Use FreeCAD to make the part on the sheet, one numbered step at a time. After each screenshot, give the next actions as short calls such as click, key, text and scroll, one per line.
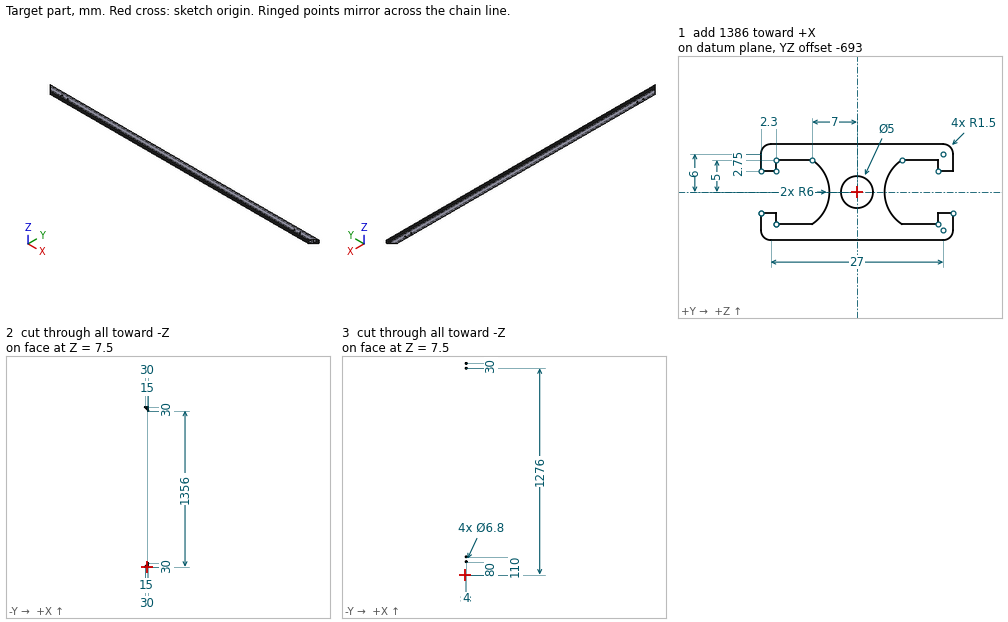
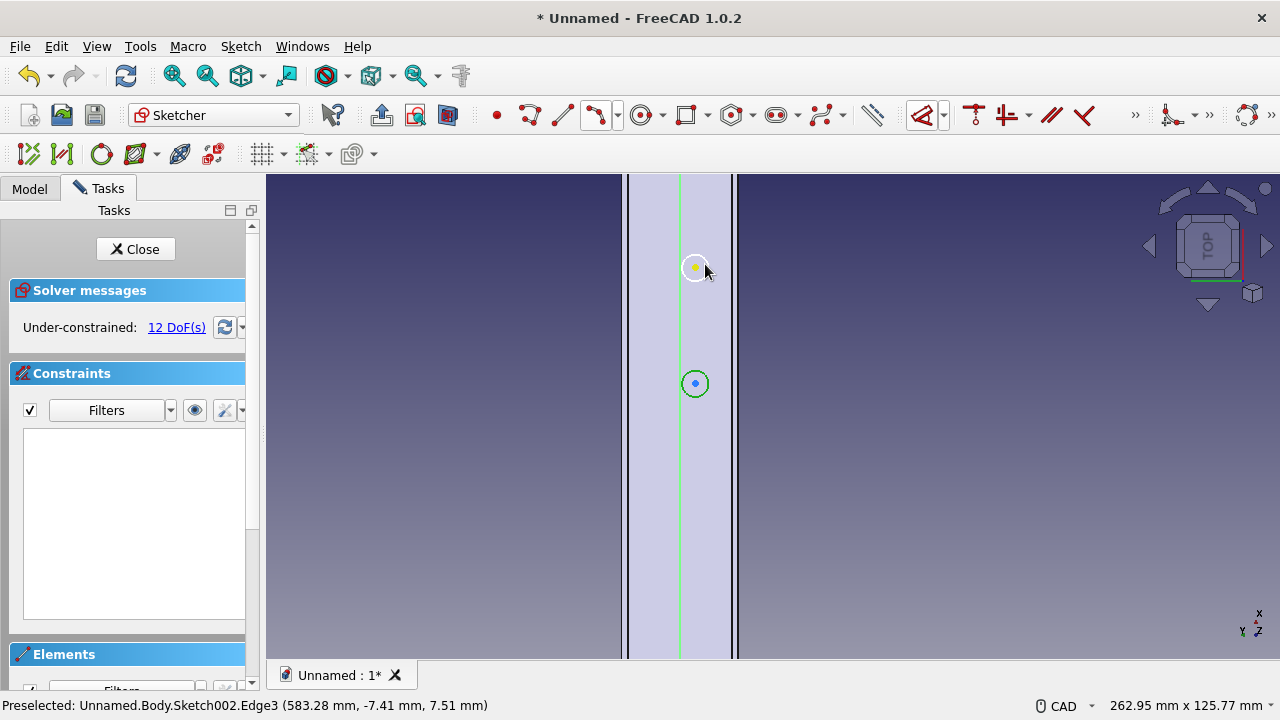
click(705, 259)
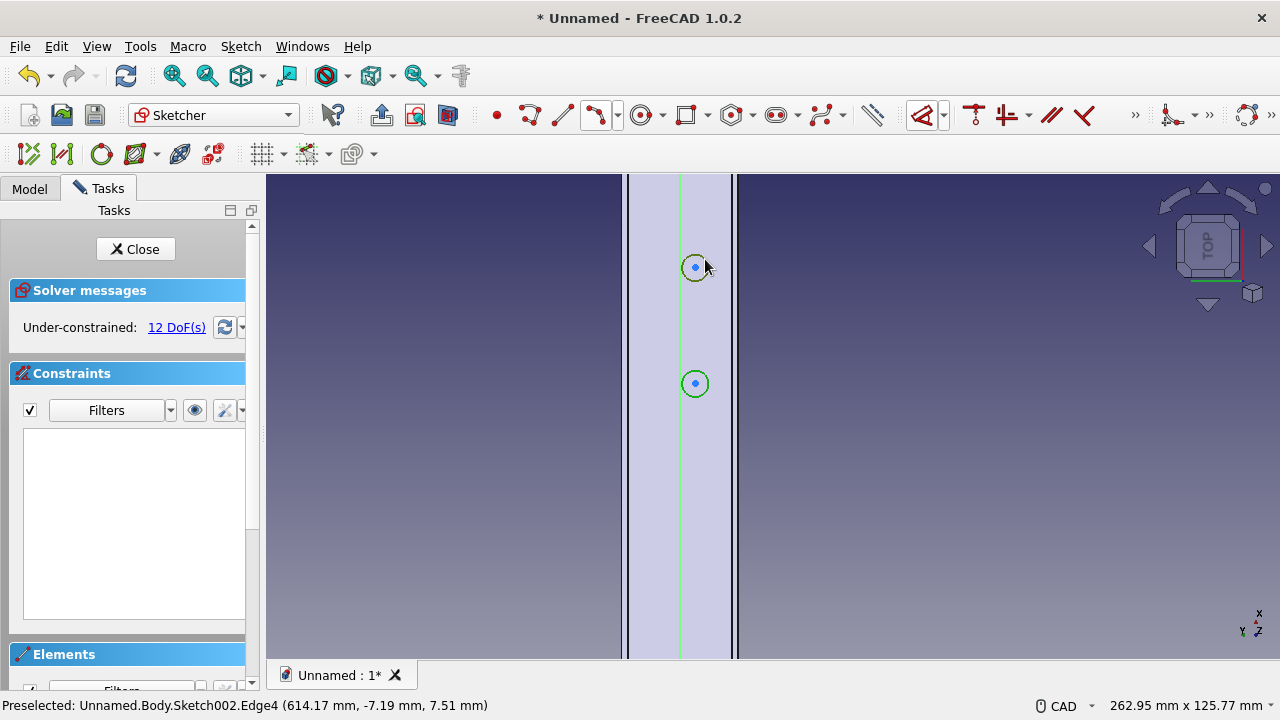
key(e)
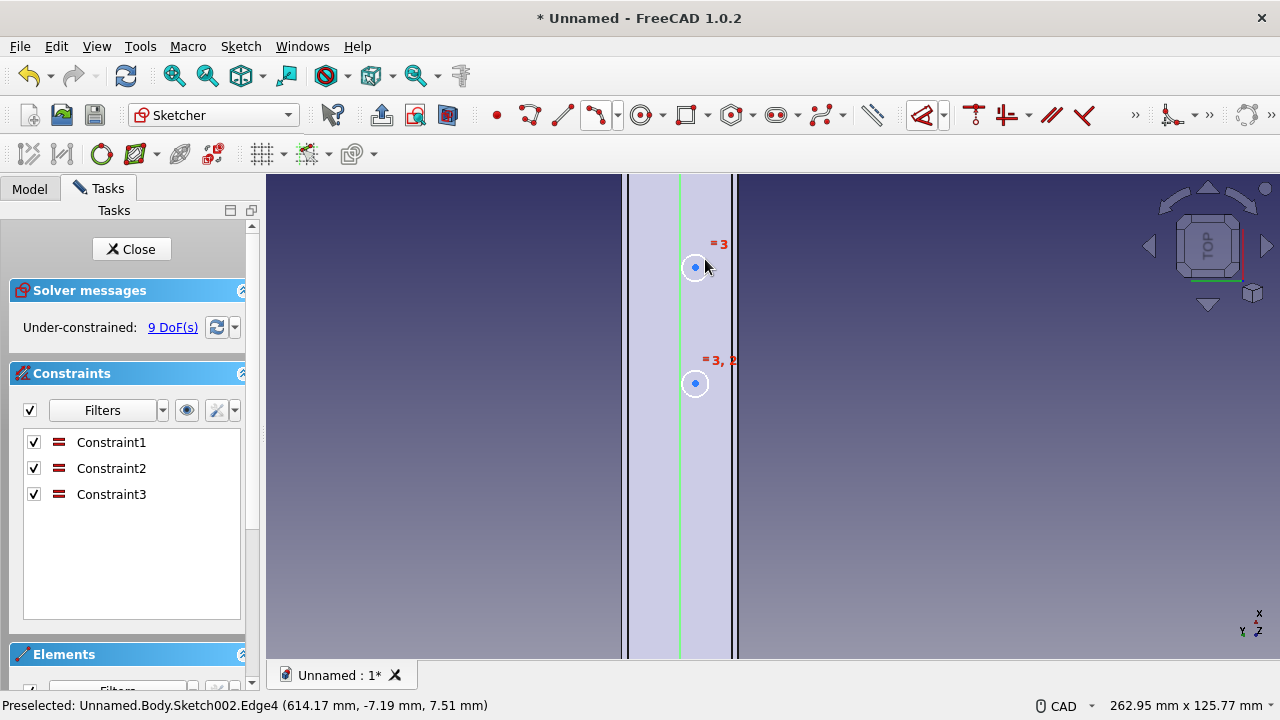
scroll(705, 264, down, 14)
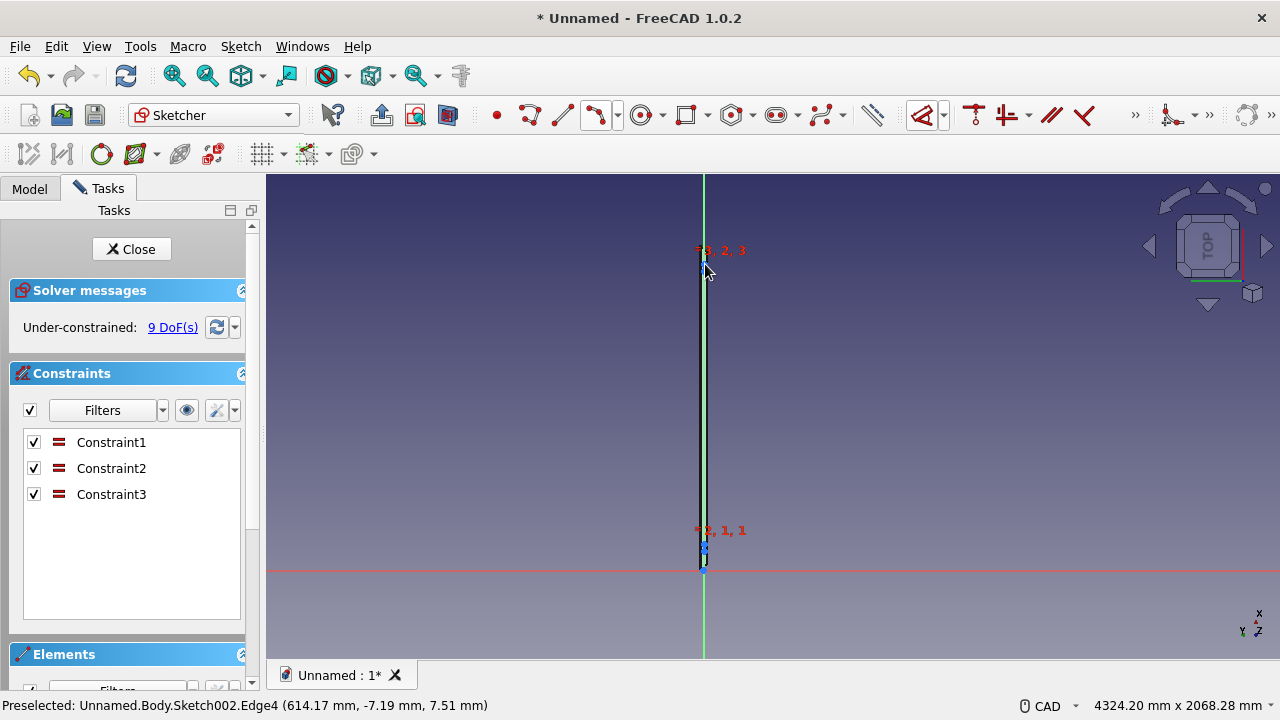
scroll(705, 552, up, 3)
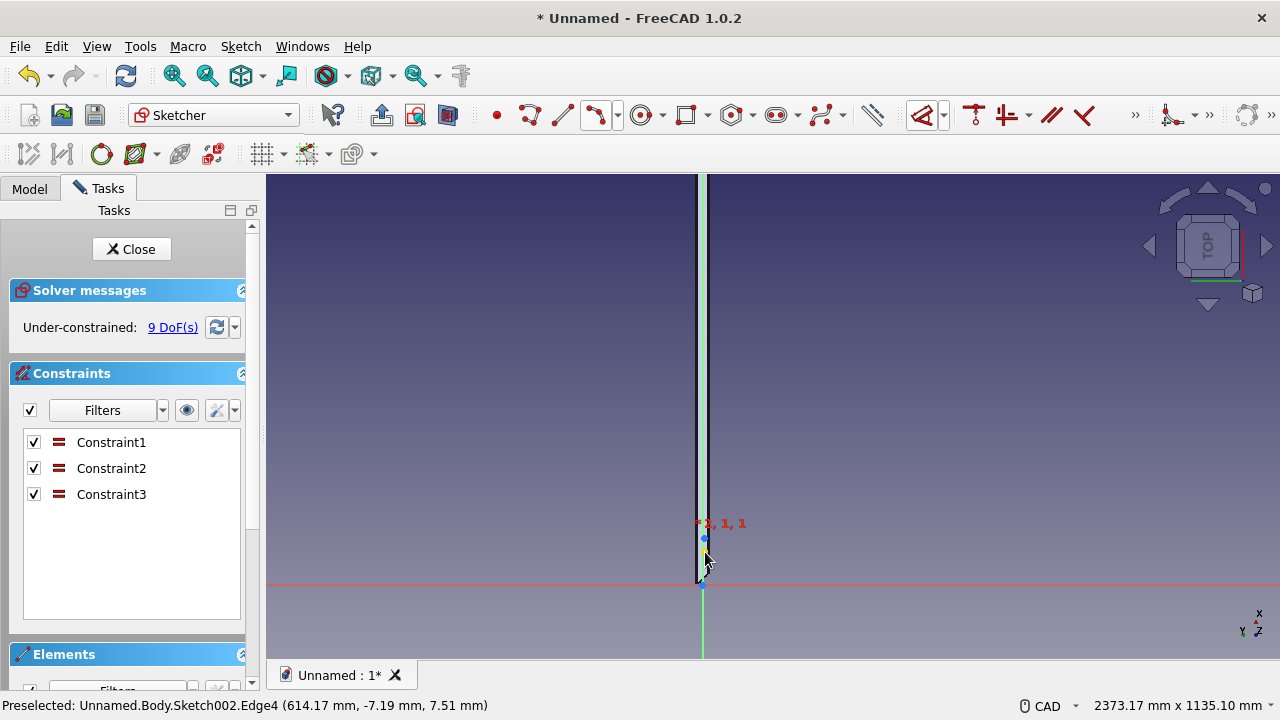
click(704, 551)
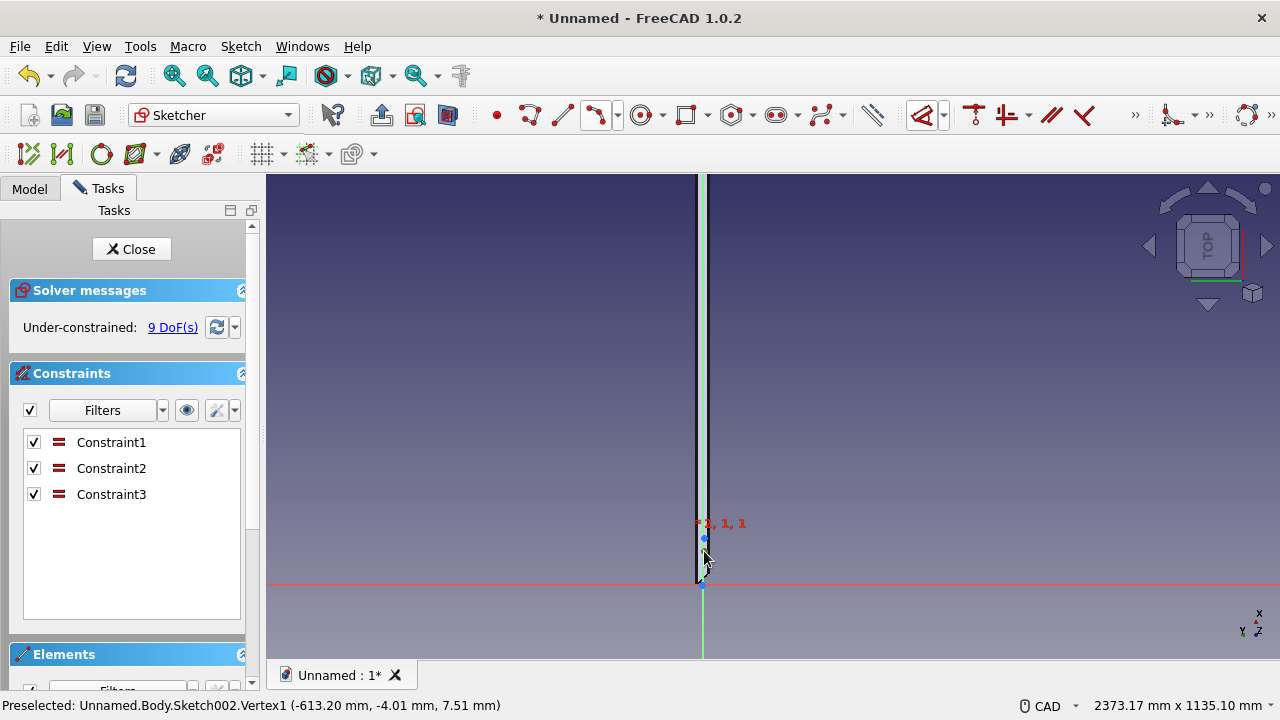
click(704, 538)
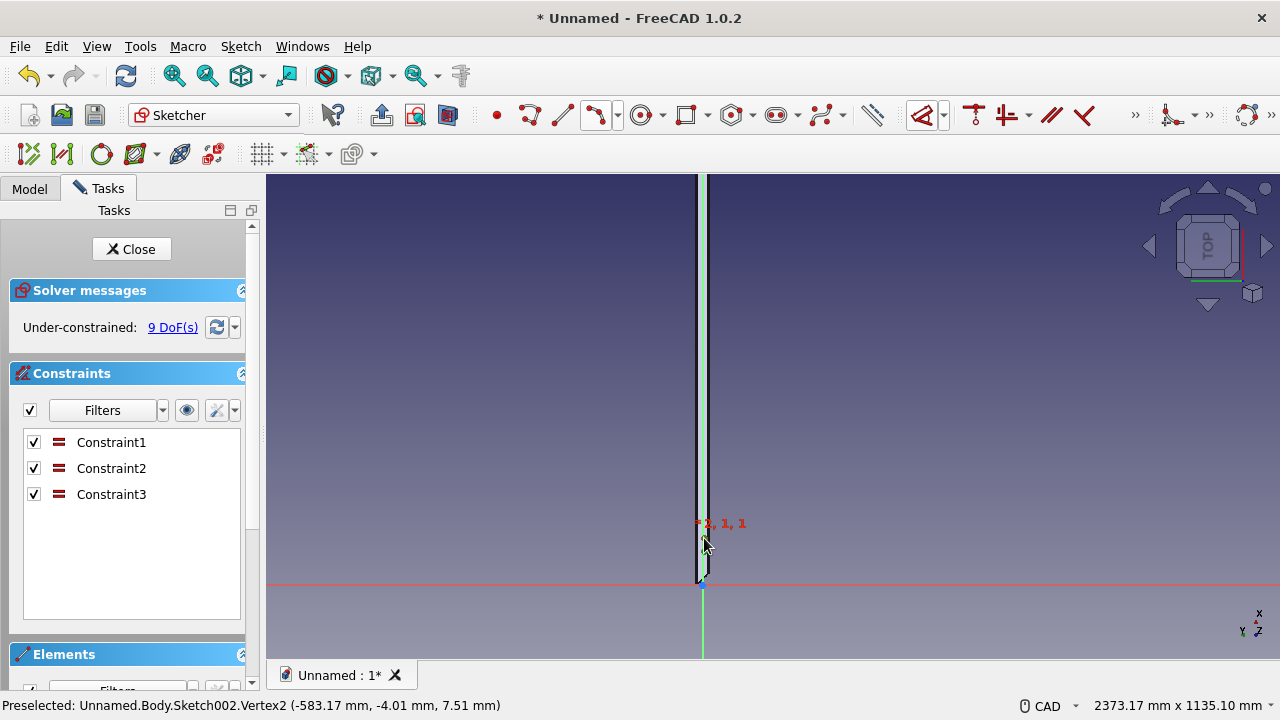
key(v)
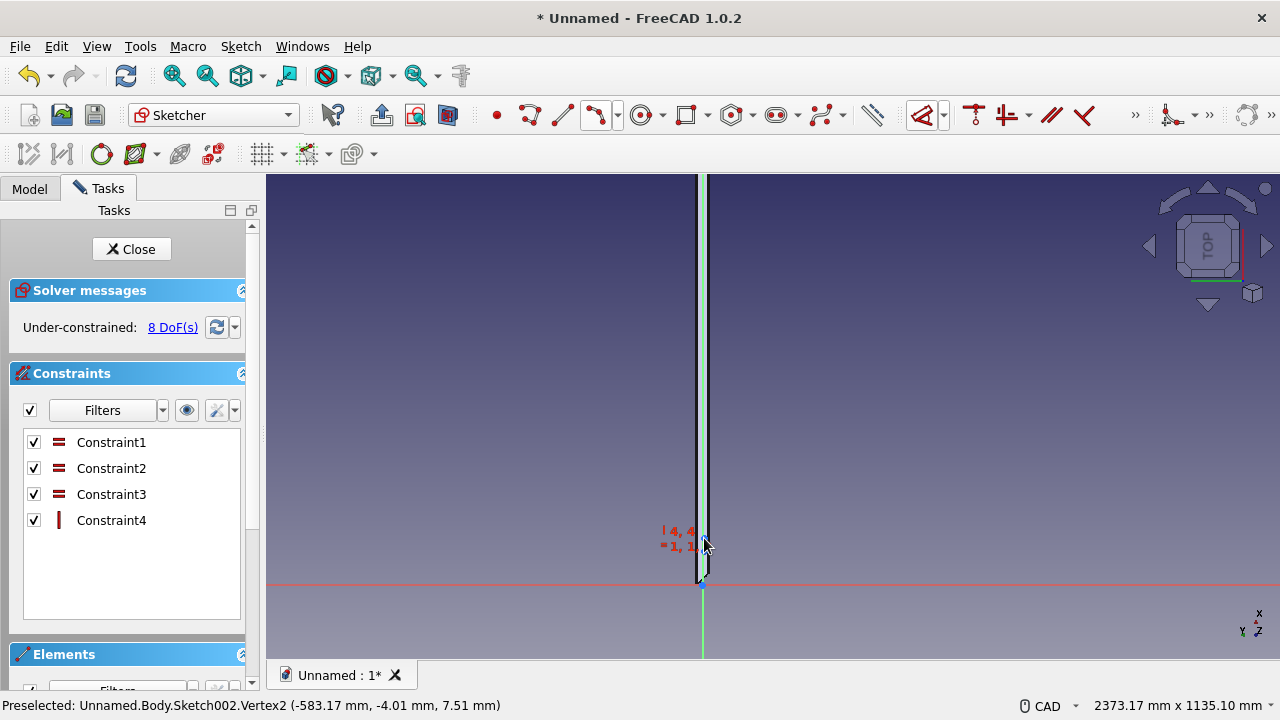
scroll(704, 538, up, 4)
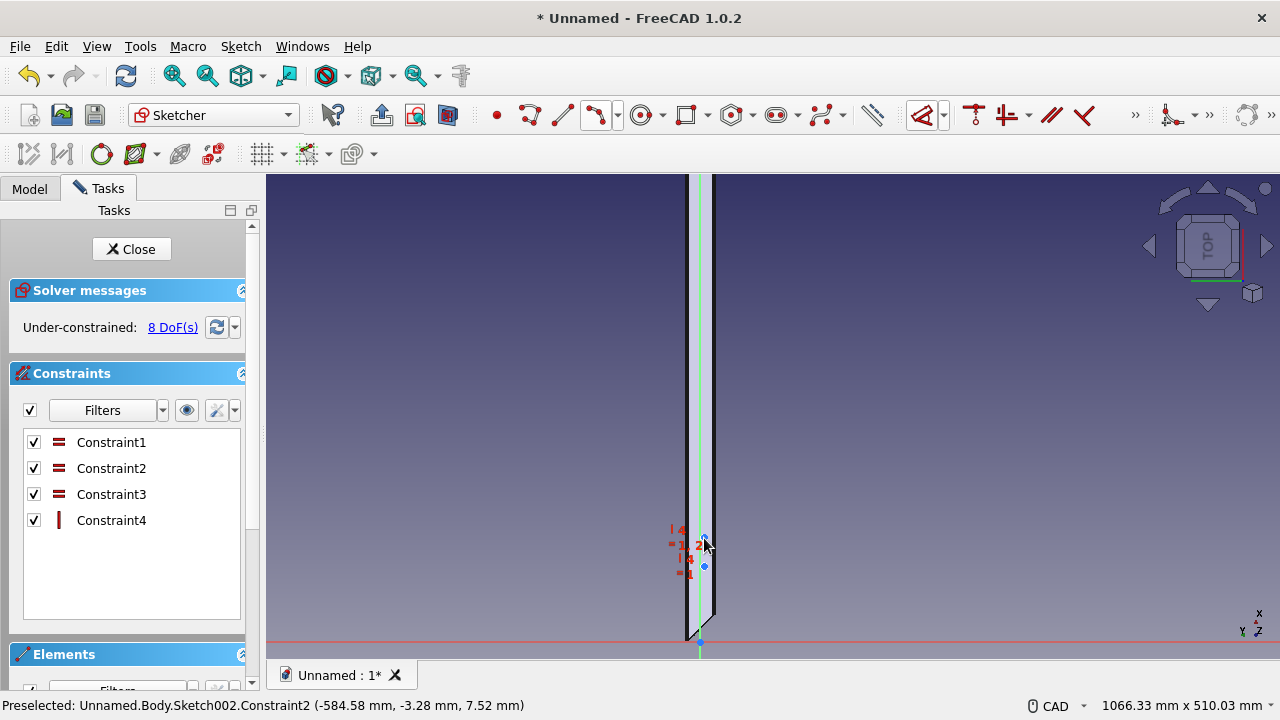
click(704, 538)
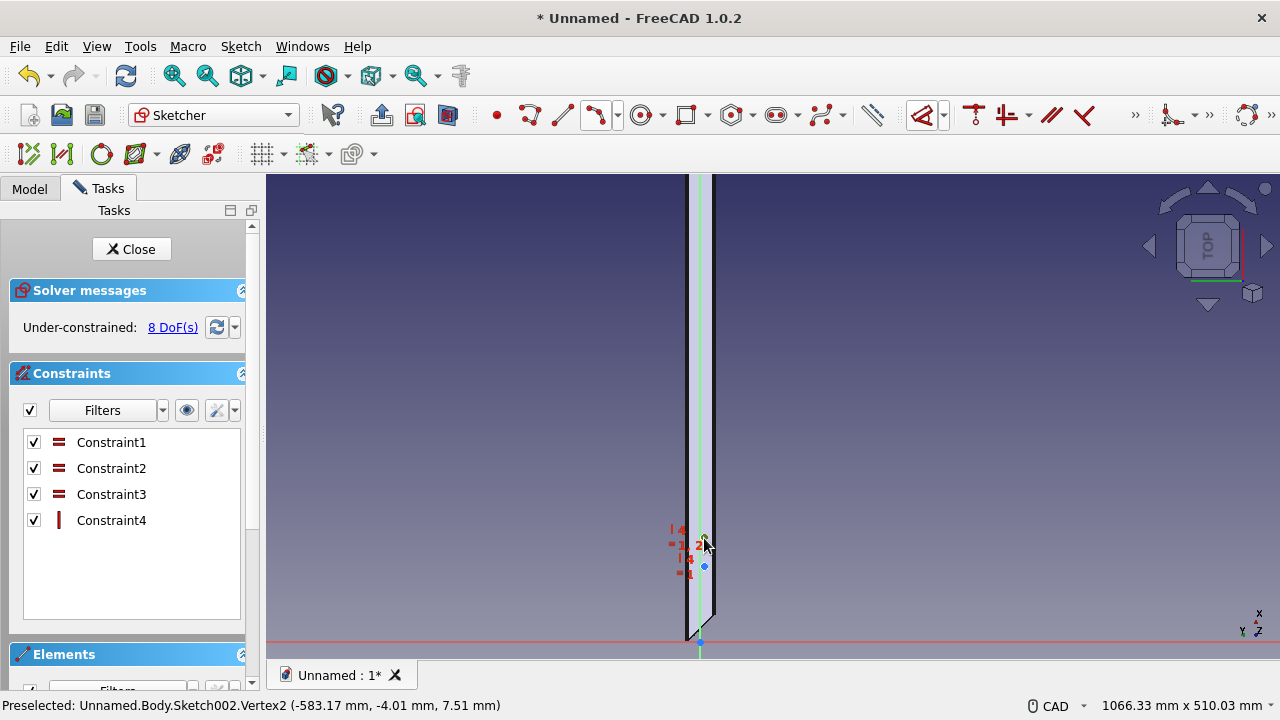
scroll(705, 546, down, 7)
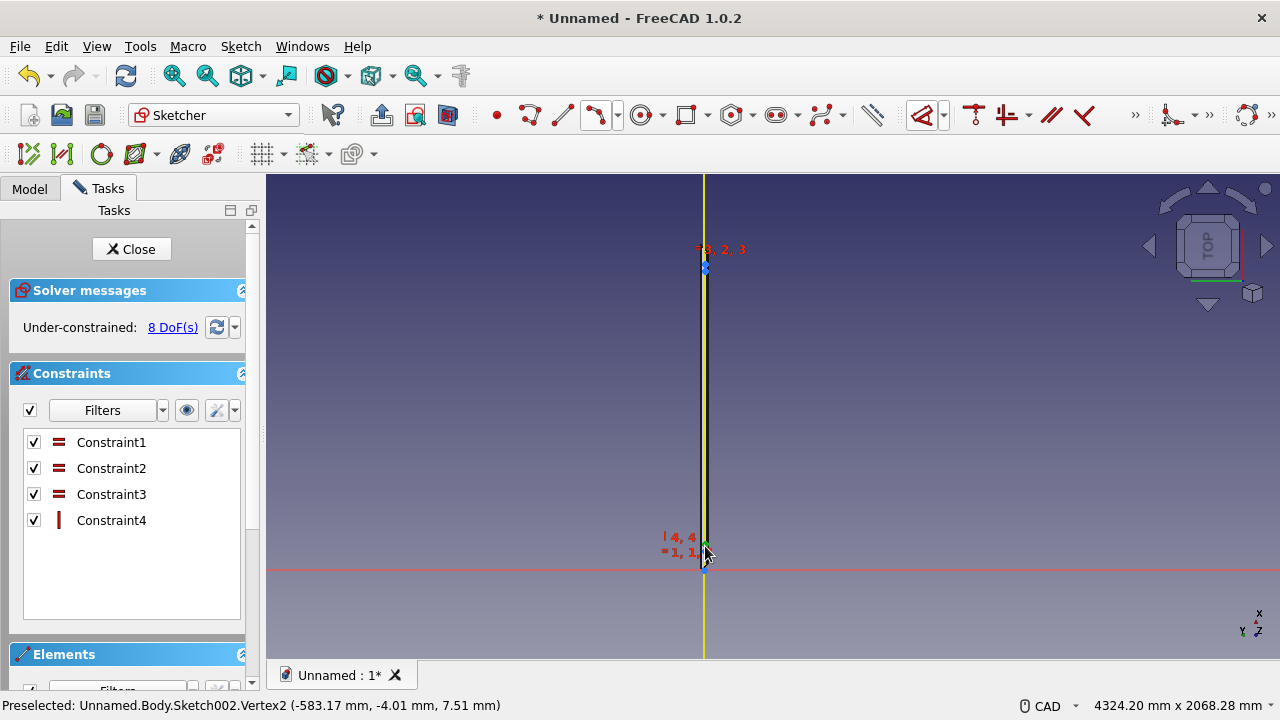
scroll(705, 271, up, 3)